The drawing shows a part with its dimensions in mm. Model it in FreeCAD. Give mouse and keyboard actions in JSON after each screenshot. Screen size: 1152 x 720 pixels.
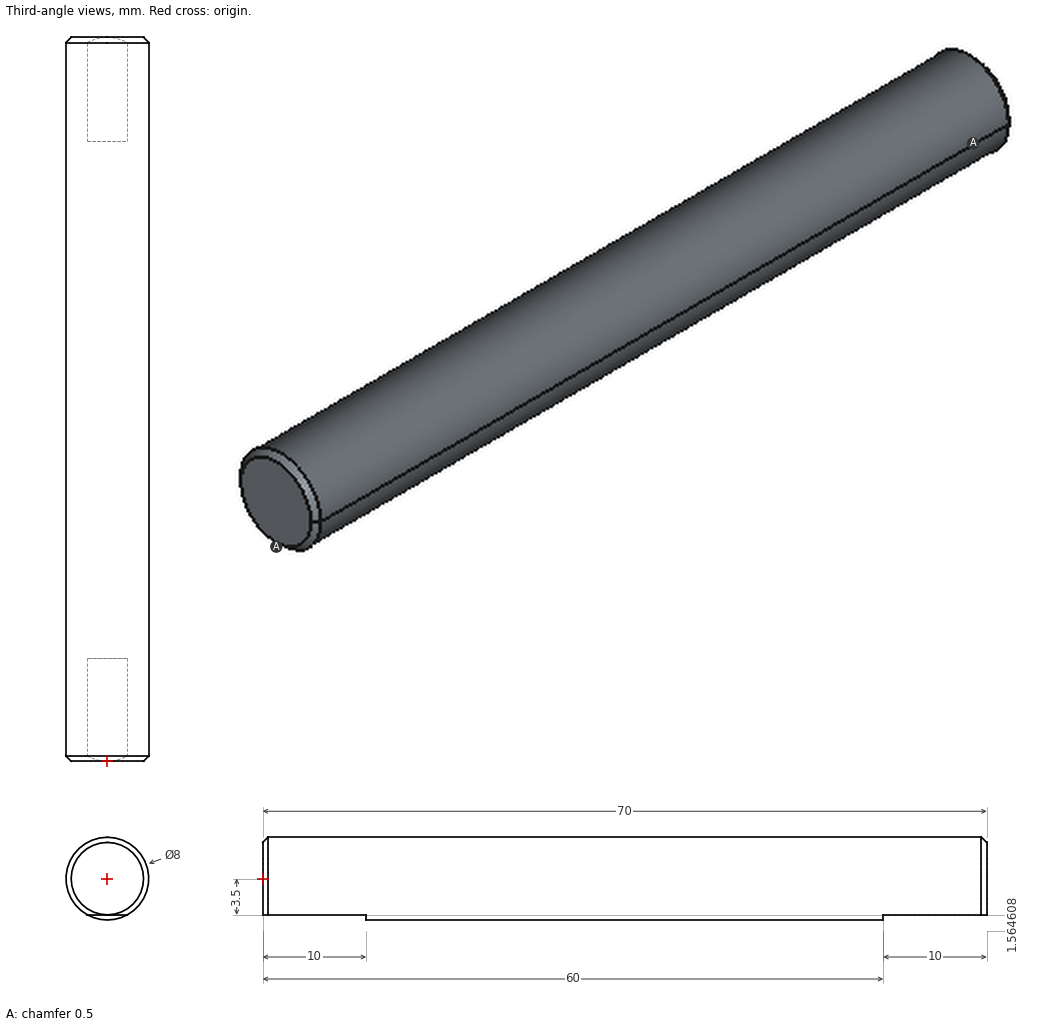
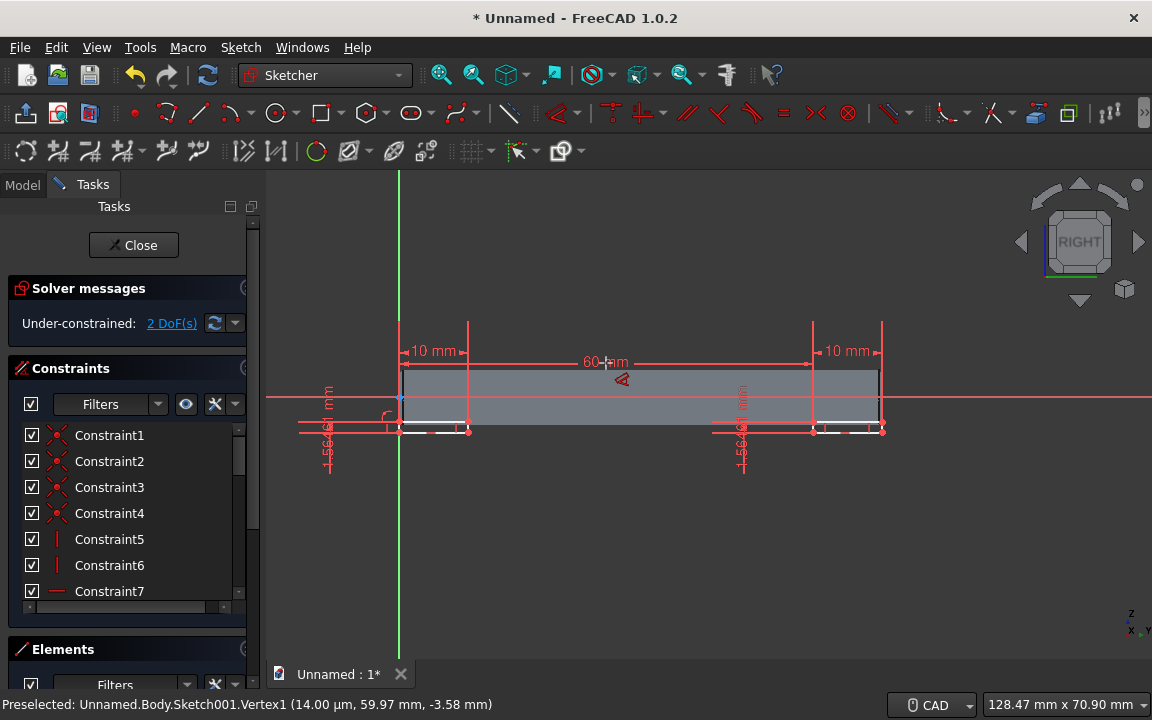
{"action": "scroll", "coordinate": [813, 422], "scroll_direction": "up", "scroll_amount": 3}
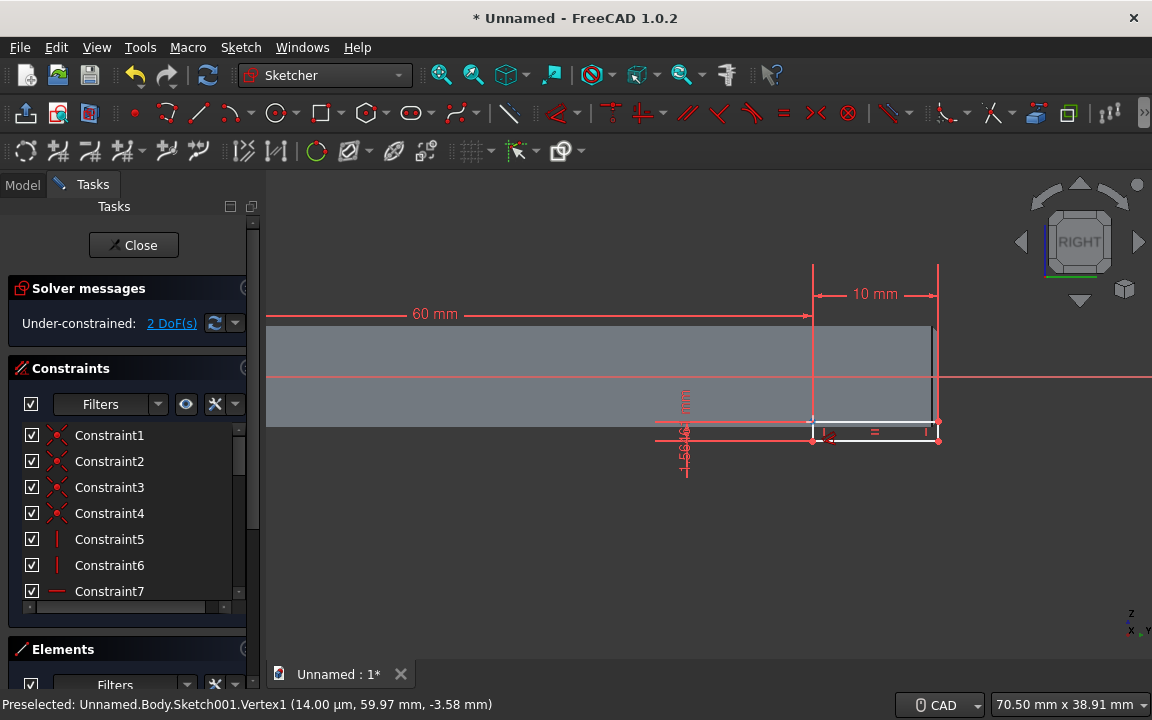
{"action": "left_click", "coordinate": [813, 422]}
{"action": "left_click", "coordinate": [847, 399]}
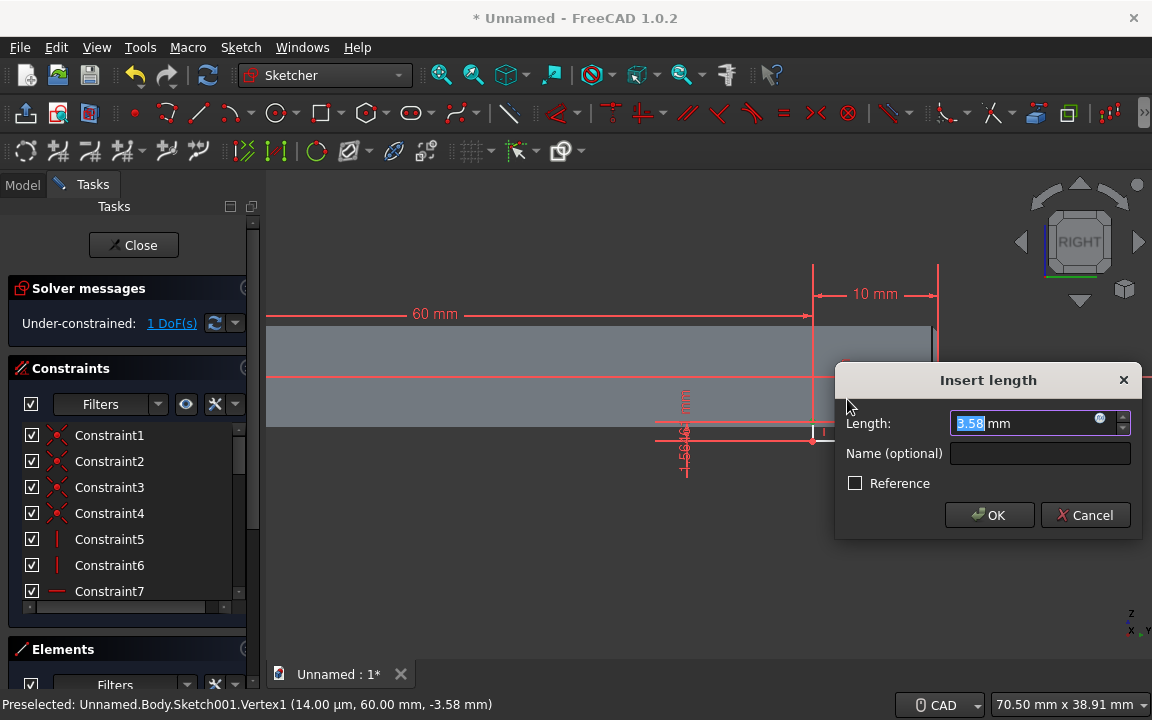
{"action": "type", "text": "3.5"}
{"action": "key", "text": "Return"}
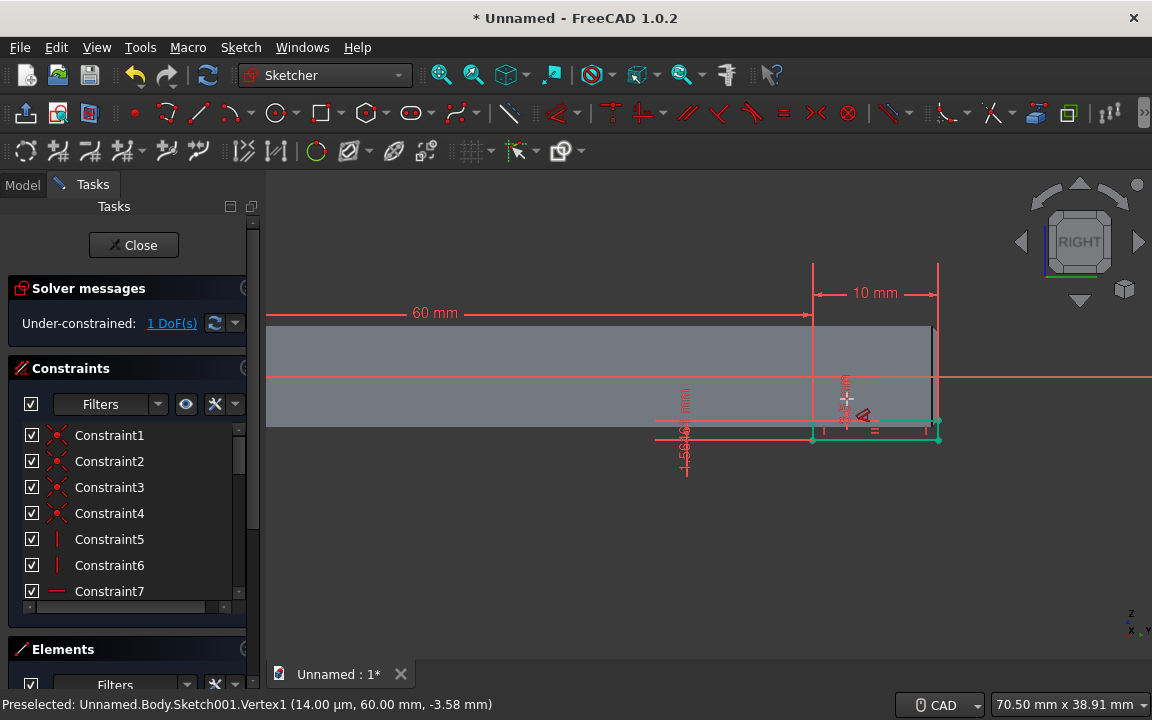
{"action": "scroll", "coordinate": [813, 422], "scroll_direction": "down", "scroll_amount": 3}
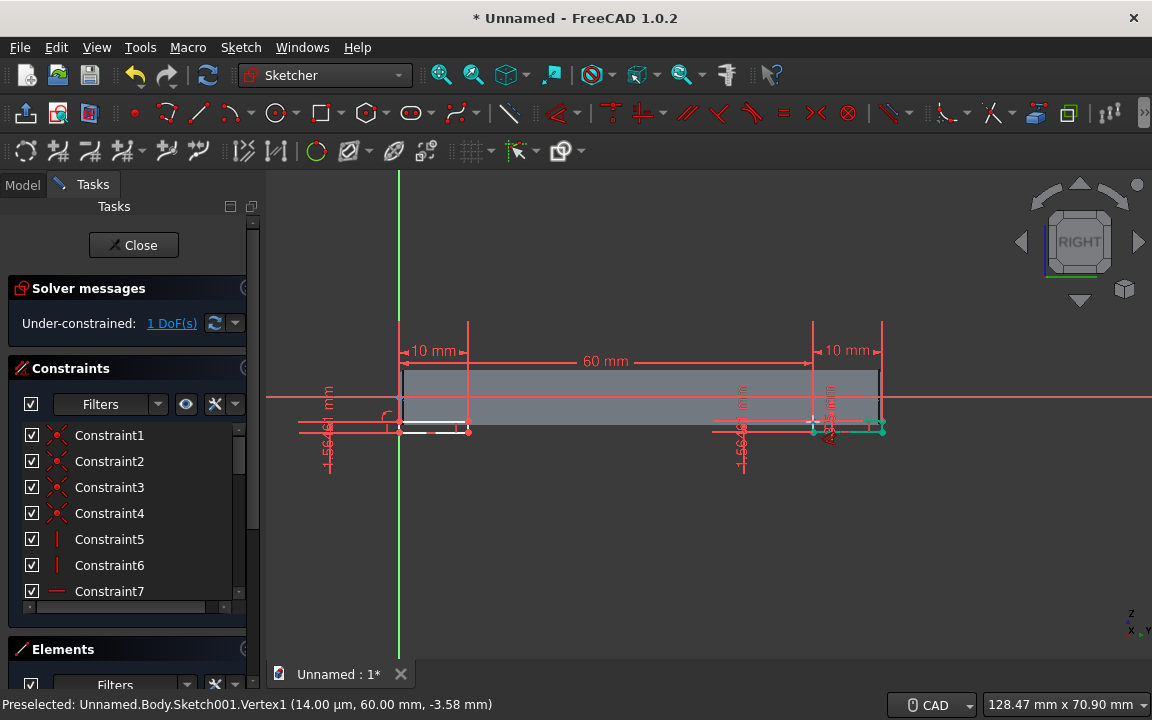
{"action": "scroll", "coordinate": [399, 422], "scroll_direction": "up", "scroll_amount": 3}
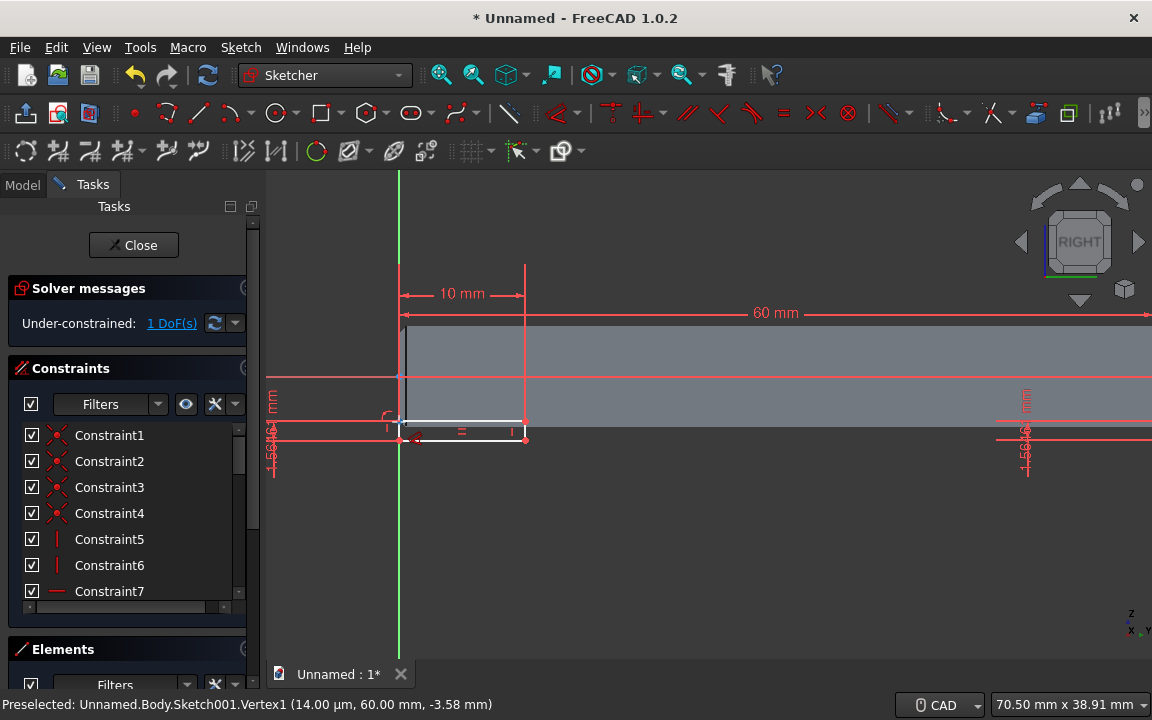
{"action": "left_click", "coordinate": [399, 421]}
{"action": "left_click", "coordinate": [365, 399]}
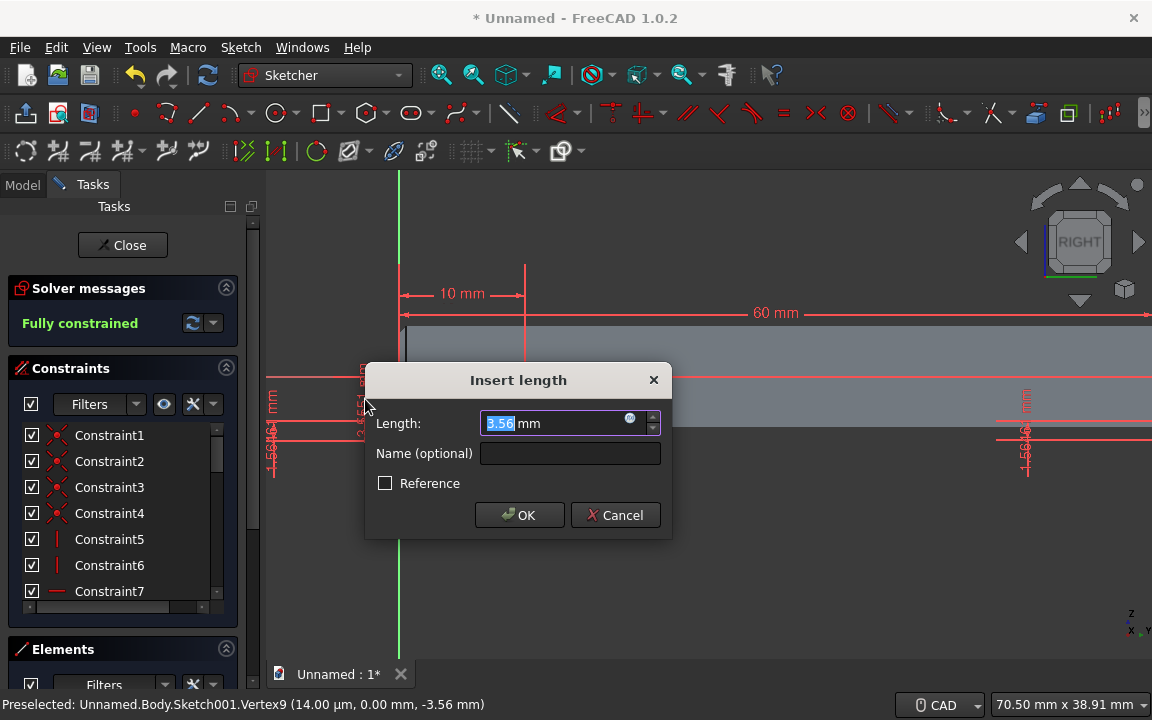
{"action": "type", "text": "3.5"}
{"action": "key", "text": "Return"}
{"action": "key", "text": "Escape"}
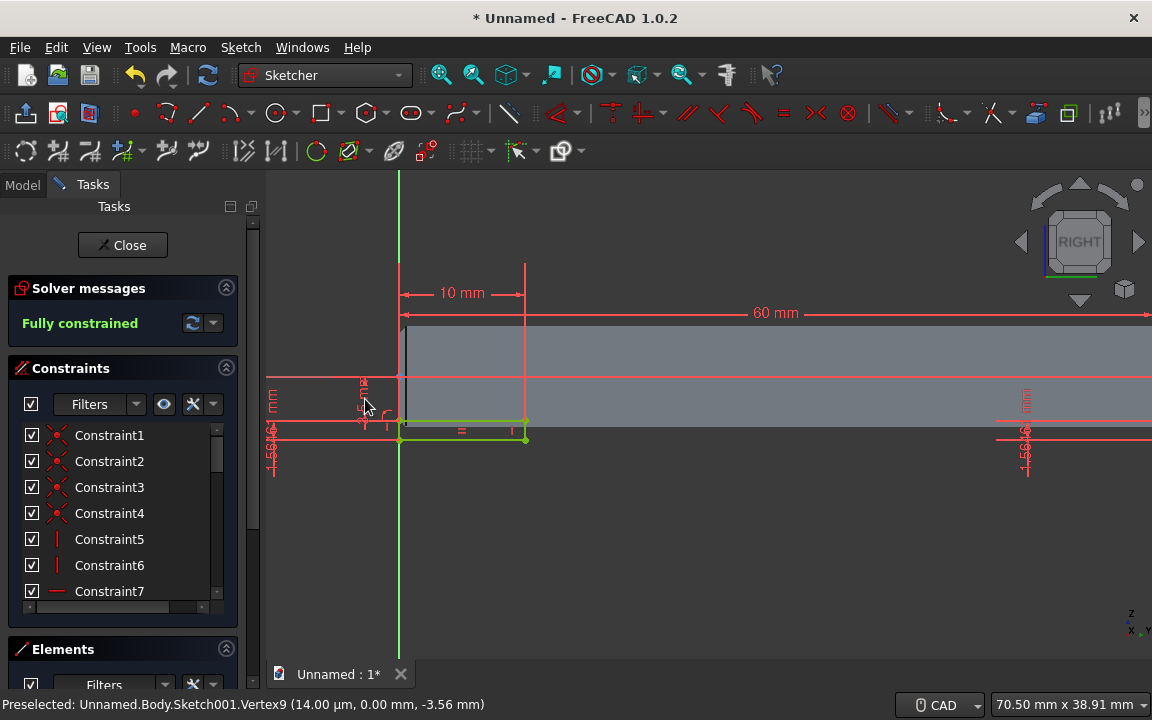
{"action": "left_click", "coordinate": [123, 245]}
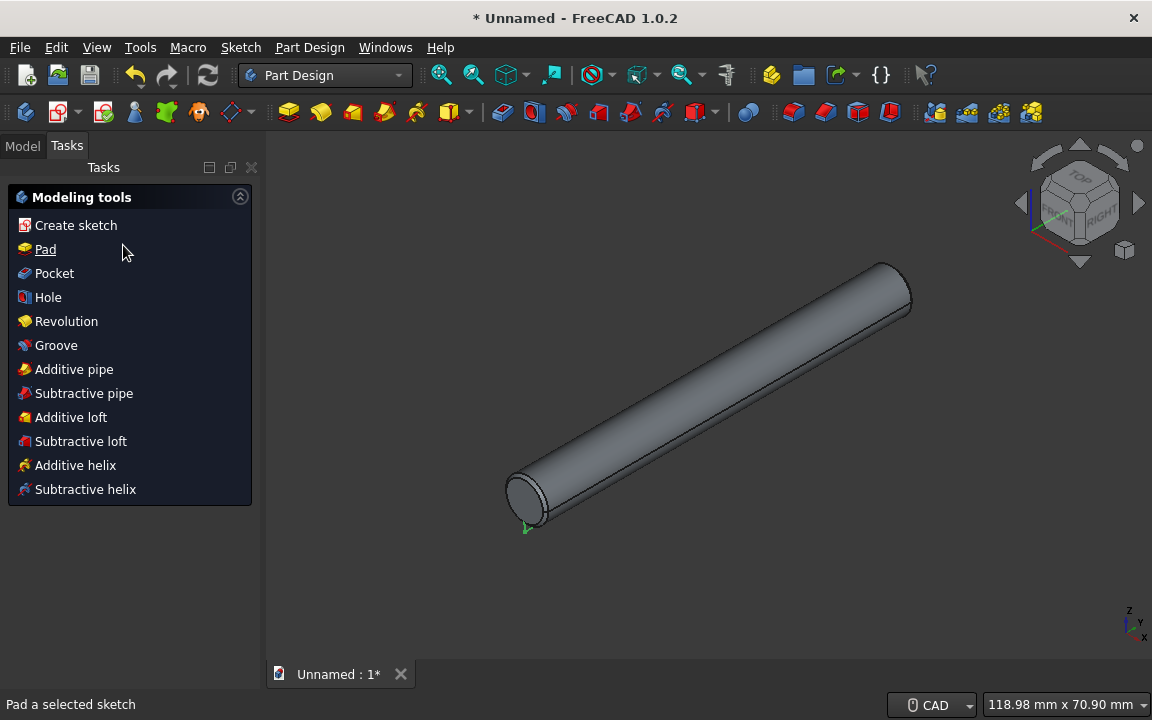
{"action": "left_click", "coordinate": [504, 112]}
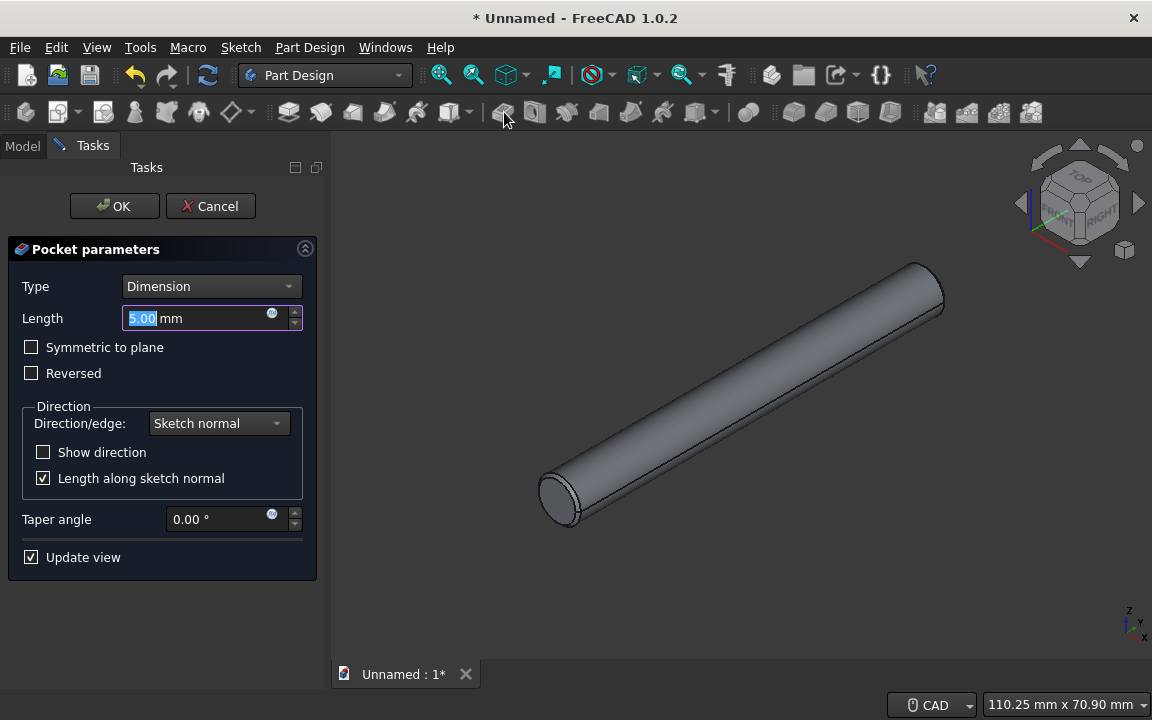
{"action": "type", "text": "10"}
{"action": "key", "text": "Tab"}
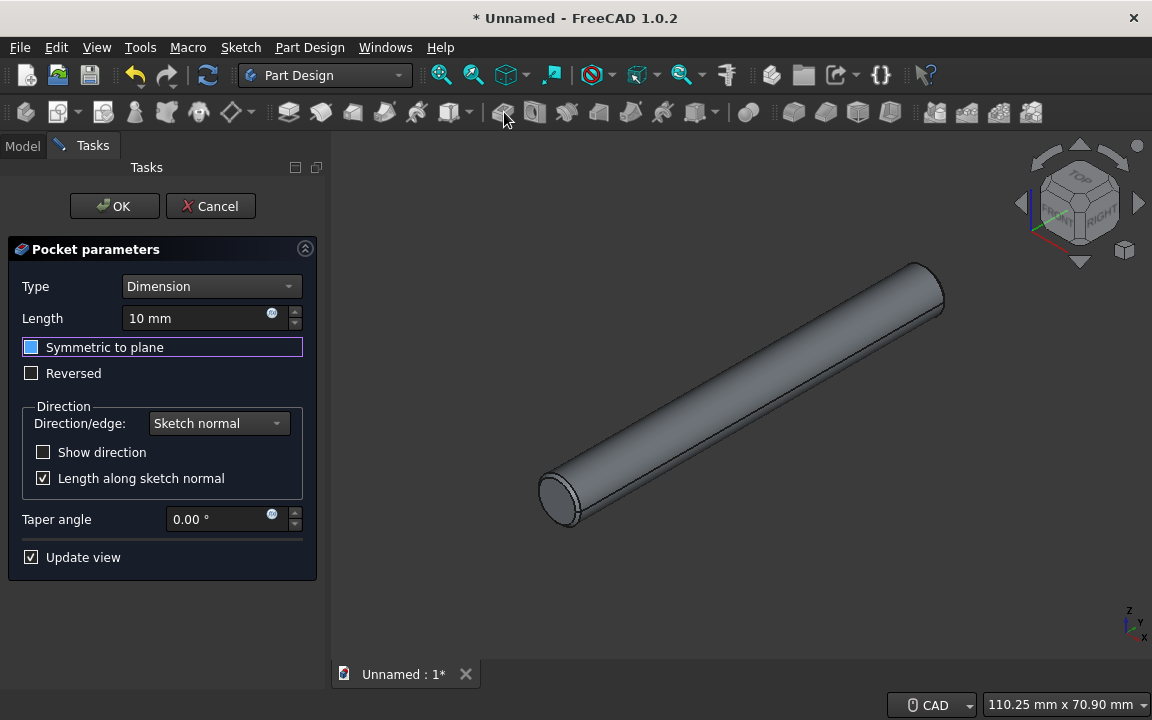
{"action": "left_click", "coordinate": [30, 347]}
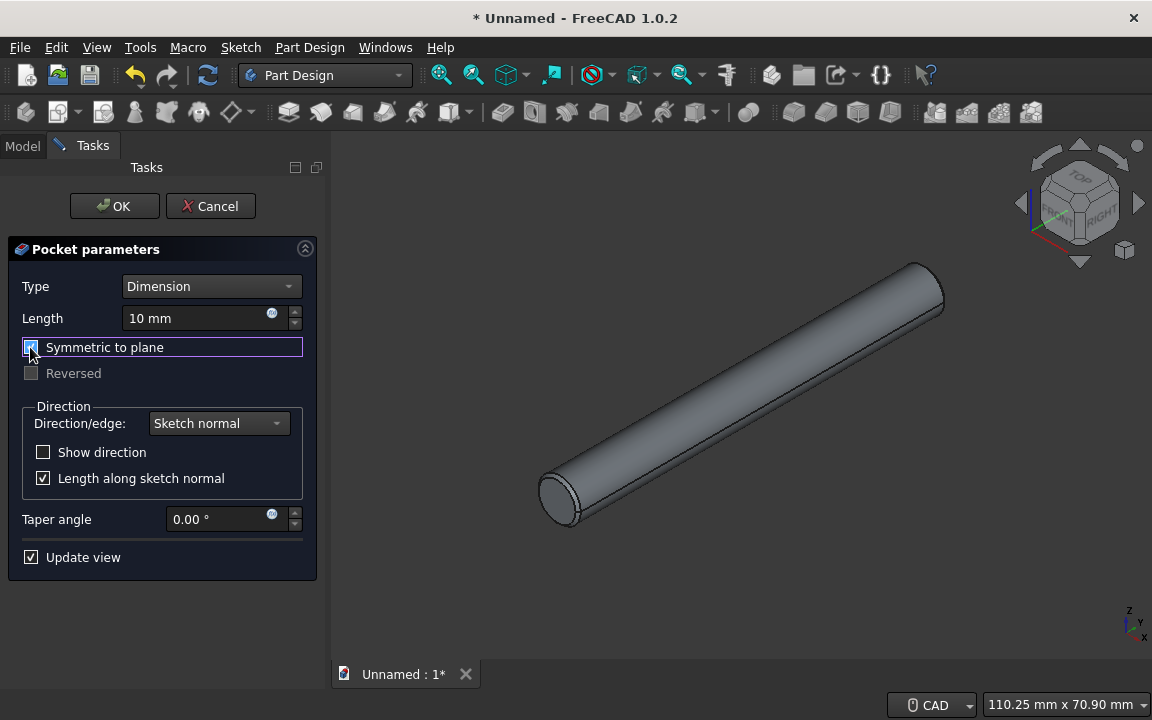
{"action": "left_click", "coordinate": [115, 206]}